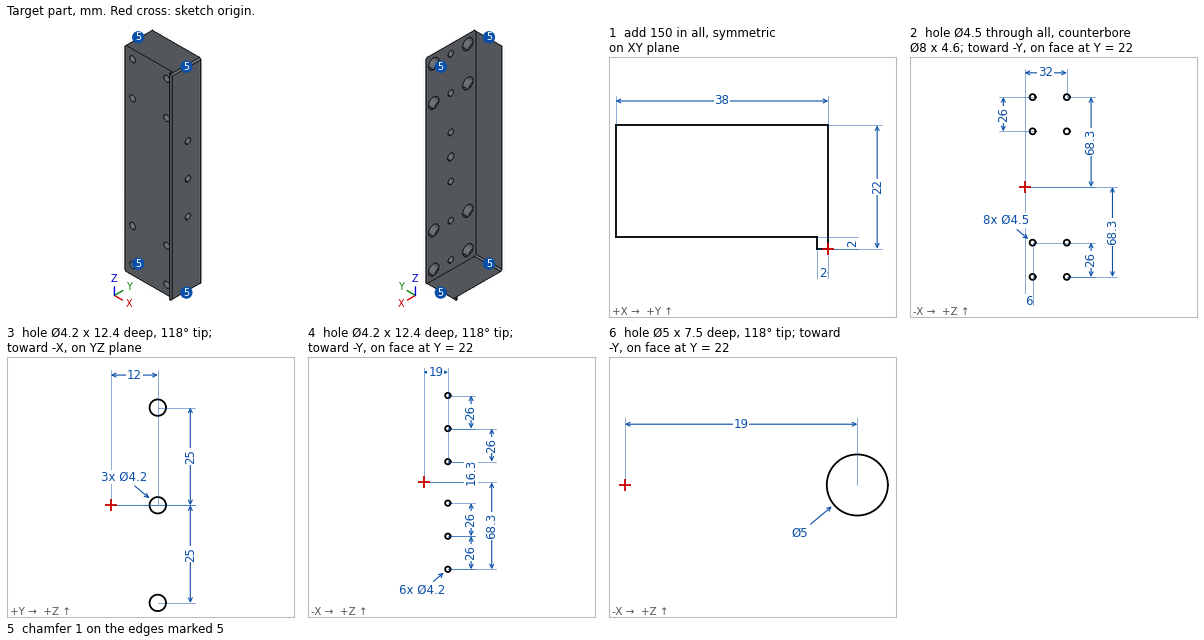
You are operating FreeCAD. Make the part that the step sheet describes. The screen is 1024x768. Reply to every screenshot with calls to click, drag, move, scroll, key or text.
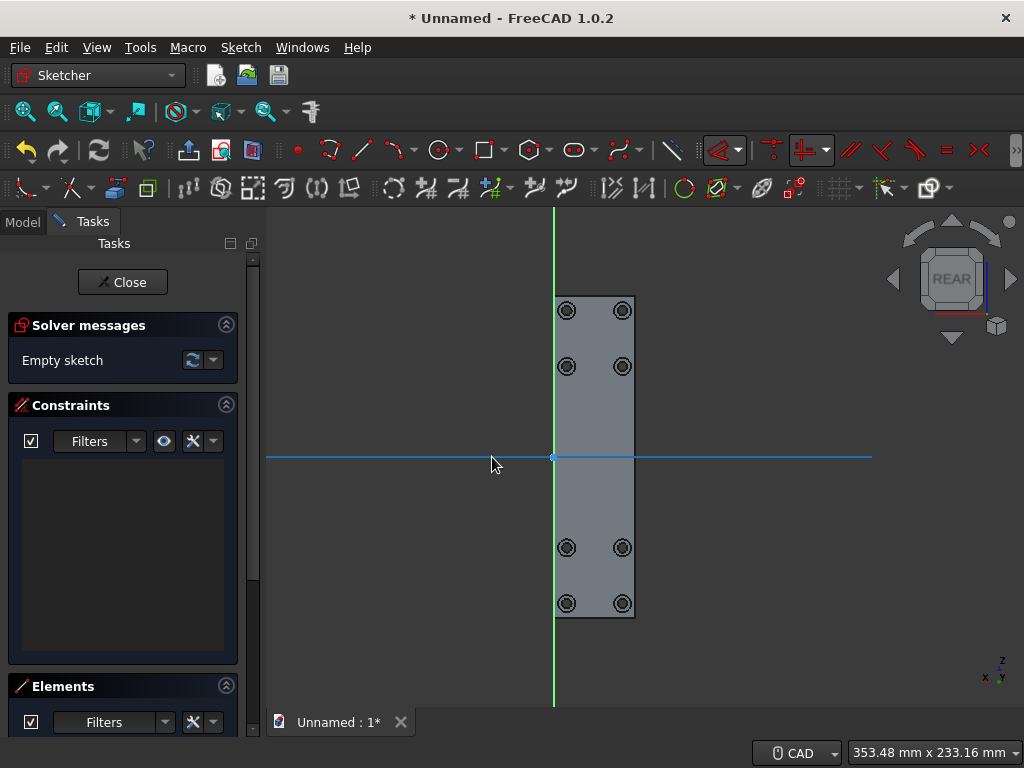
click(440, 150)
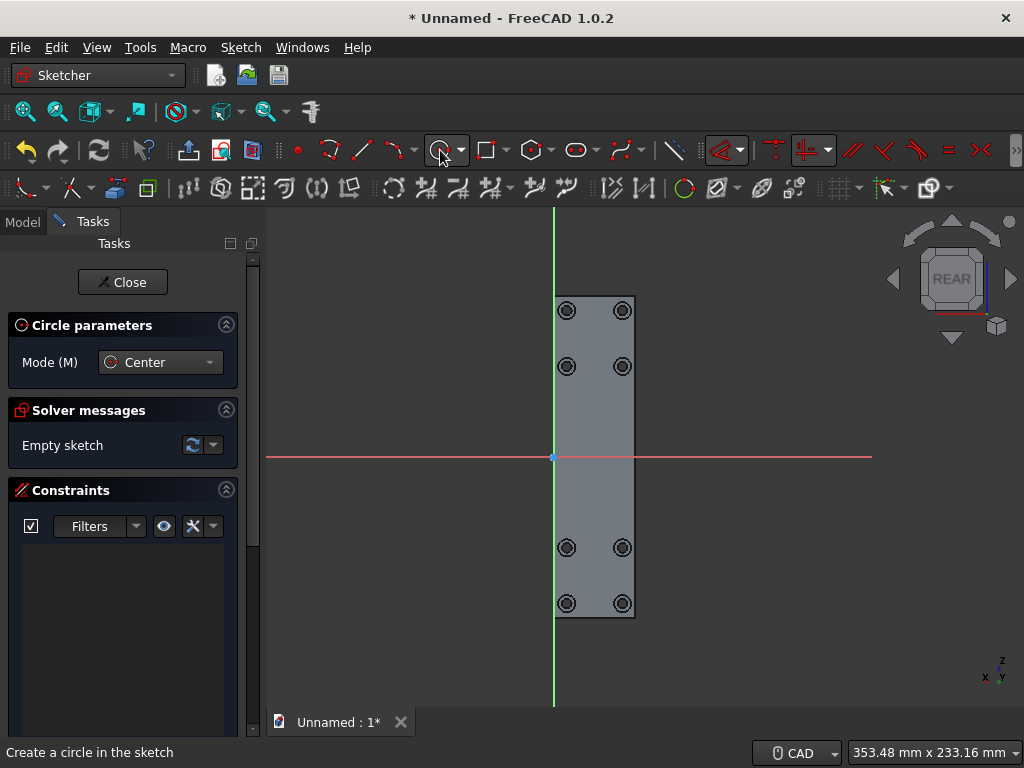
scroll(595, 422, up, 9)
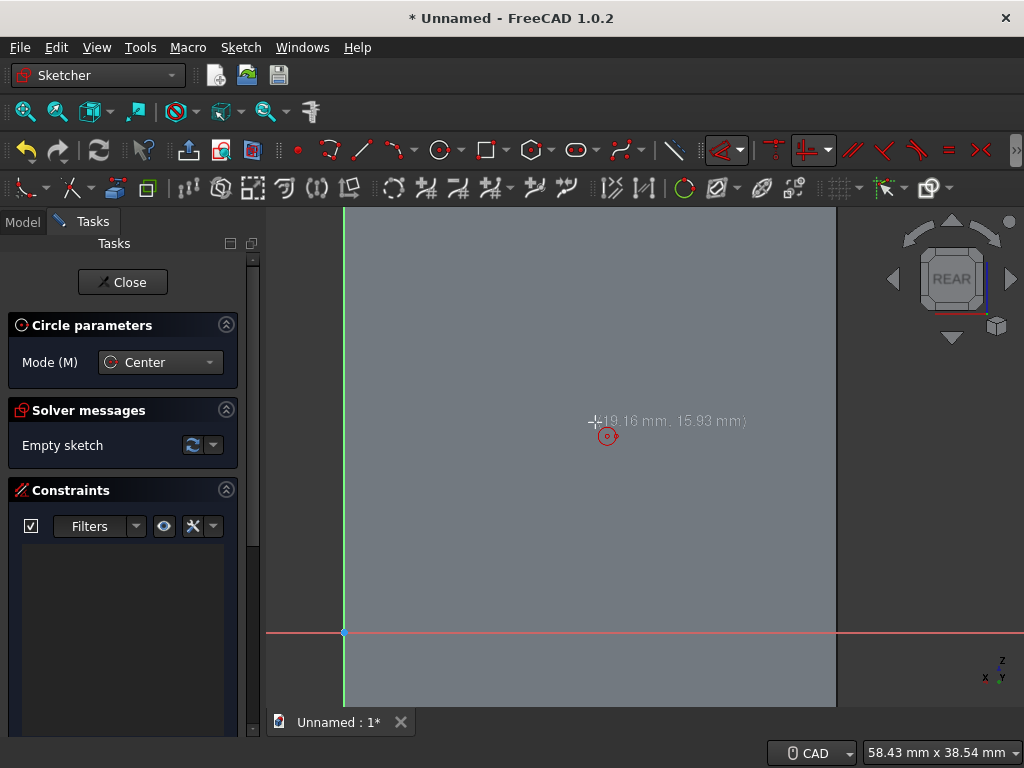
scroll(595, 422, down, 9)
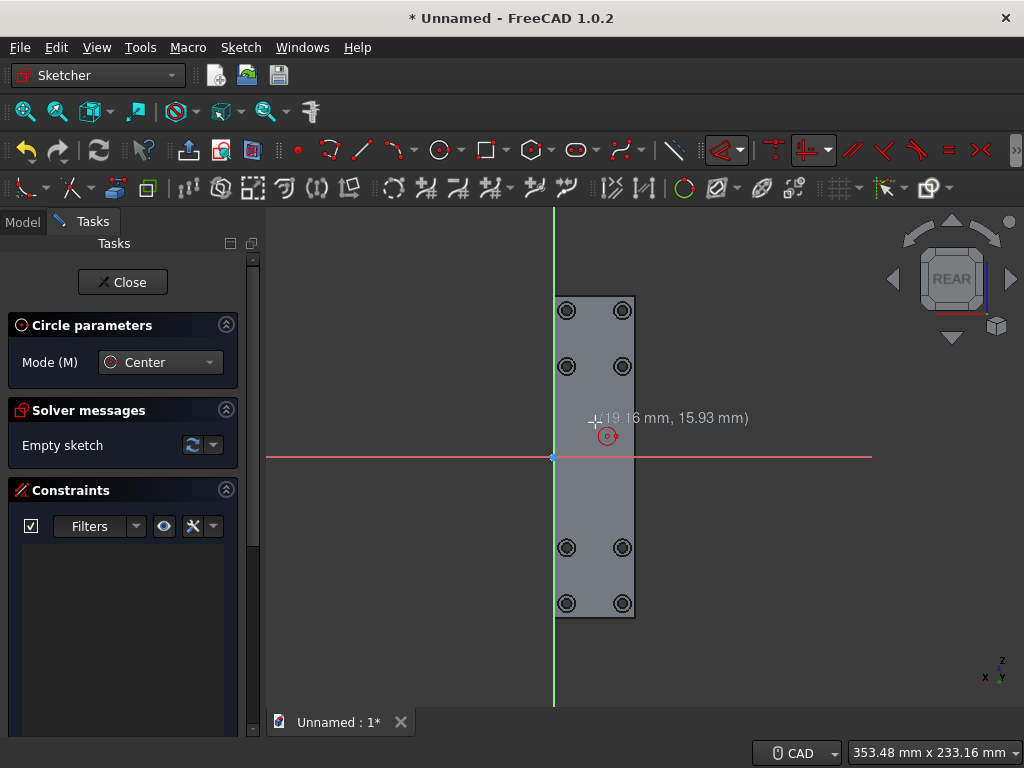
click(595, 422)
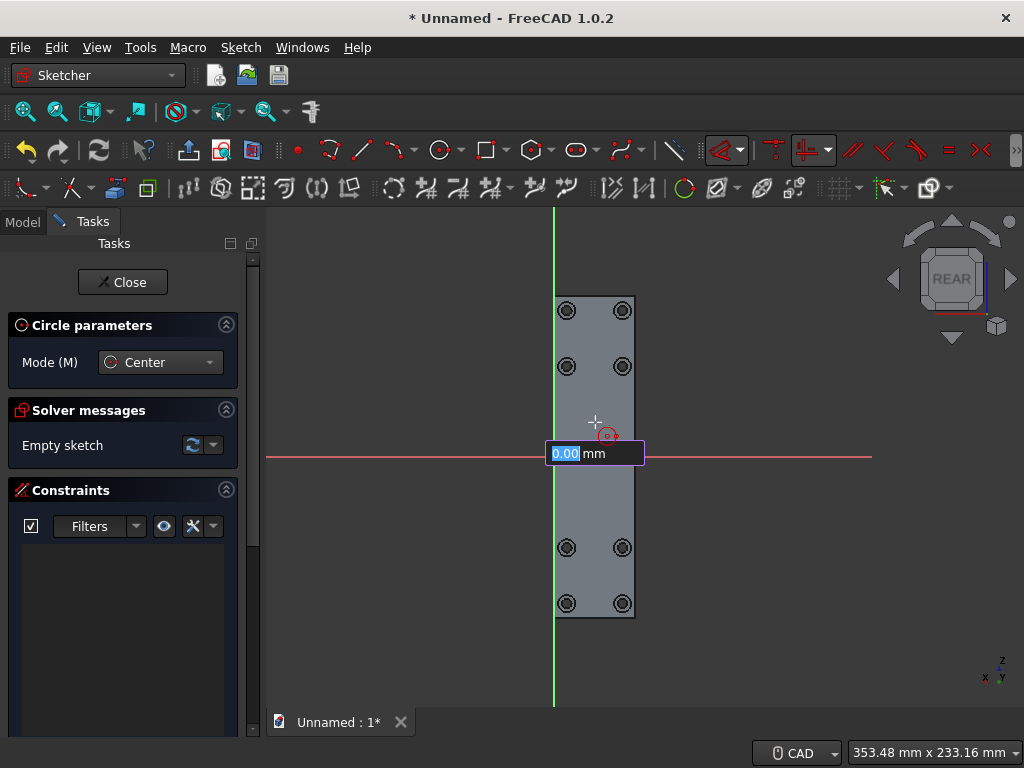
scroll(598, 419, up, 7)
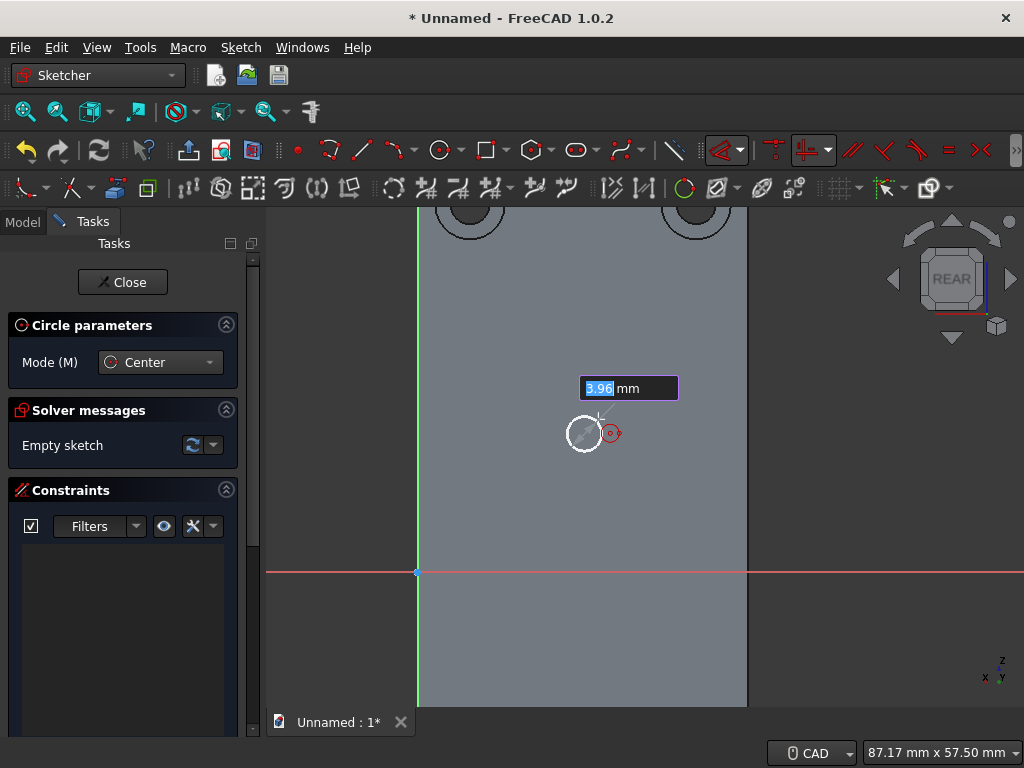
click(596, 418)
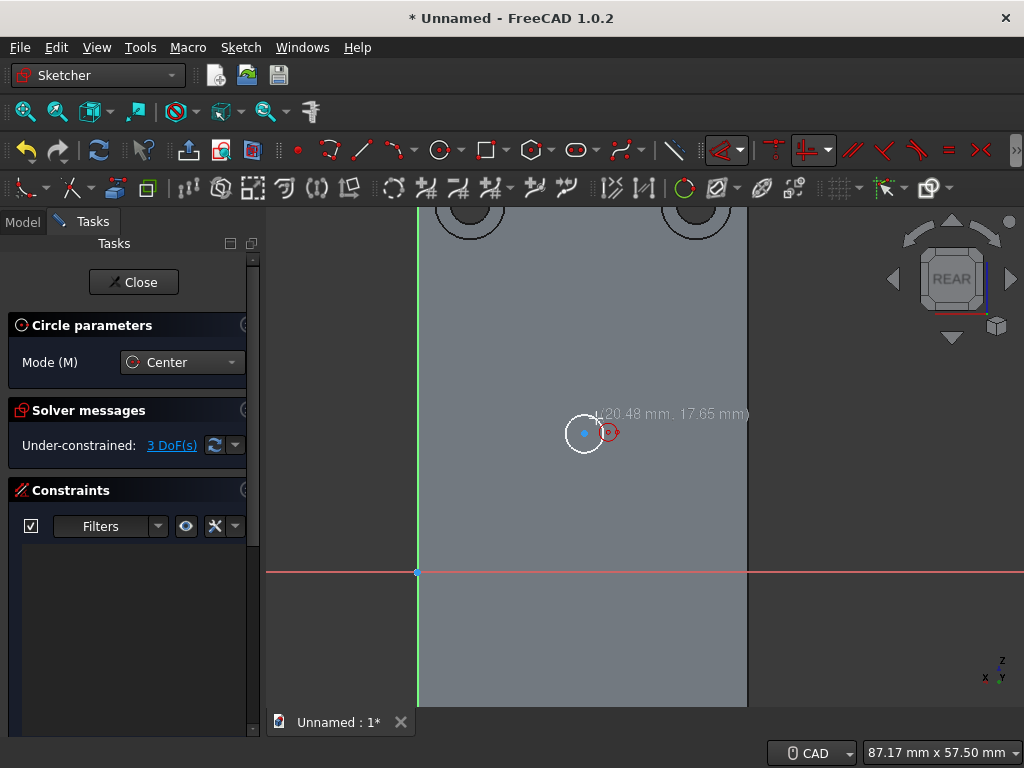
scroll(598, 419, down, 7)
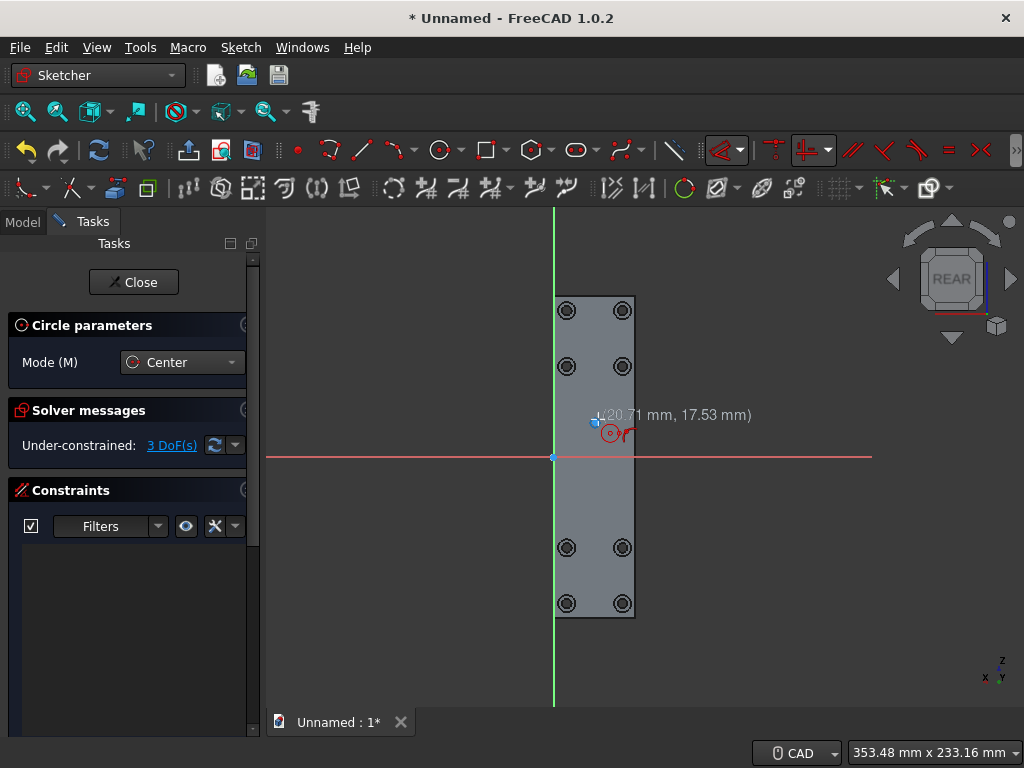
scroll(595, 604, up, 9)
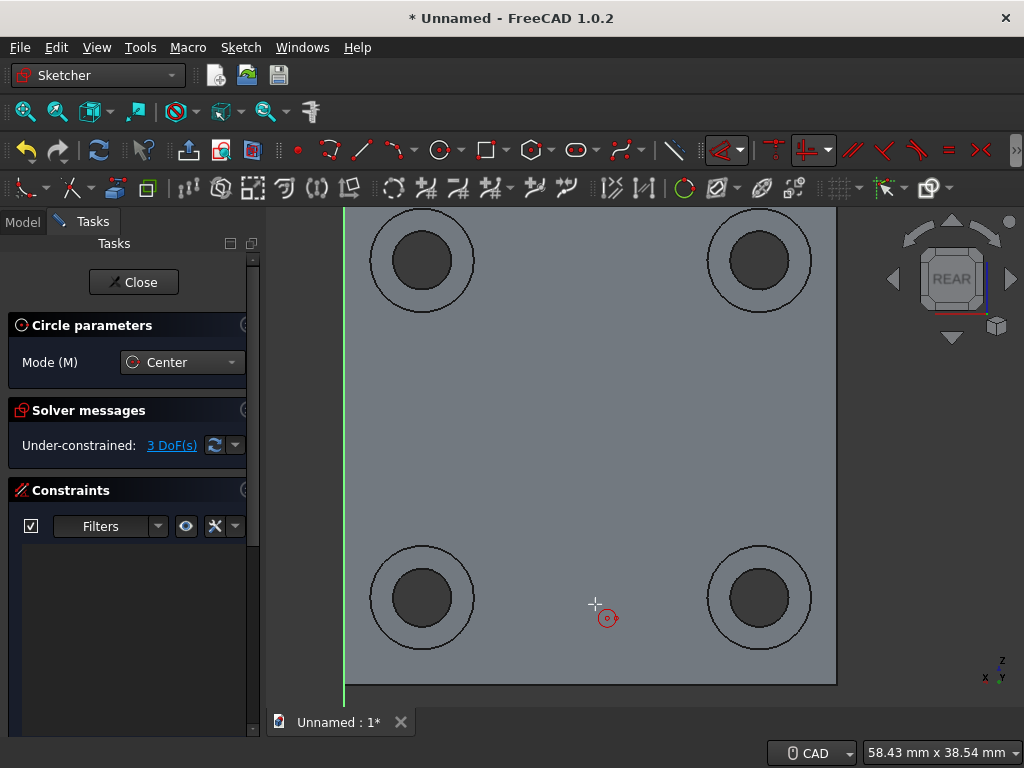
scroll(595, 605, down, 9)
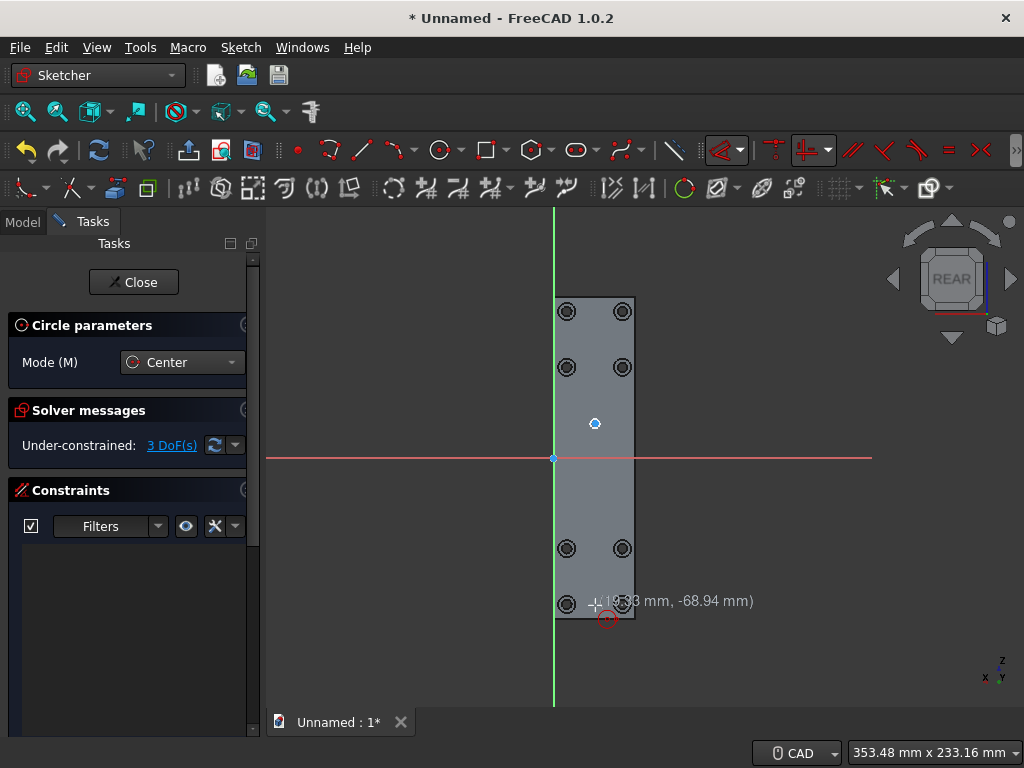
click(595, 604)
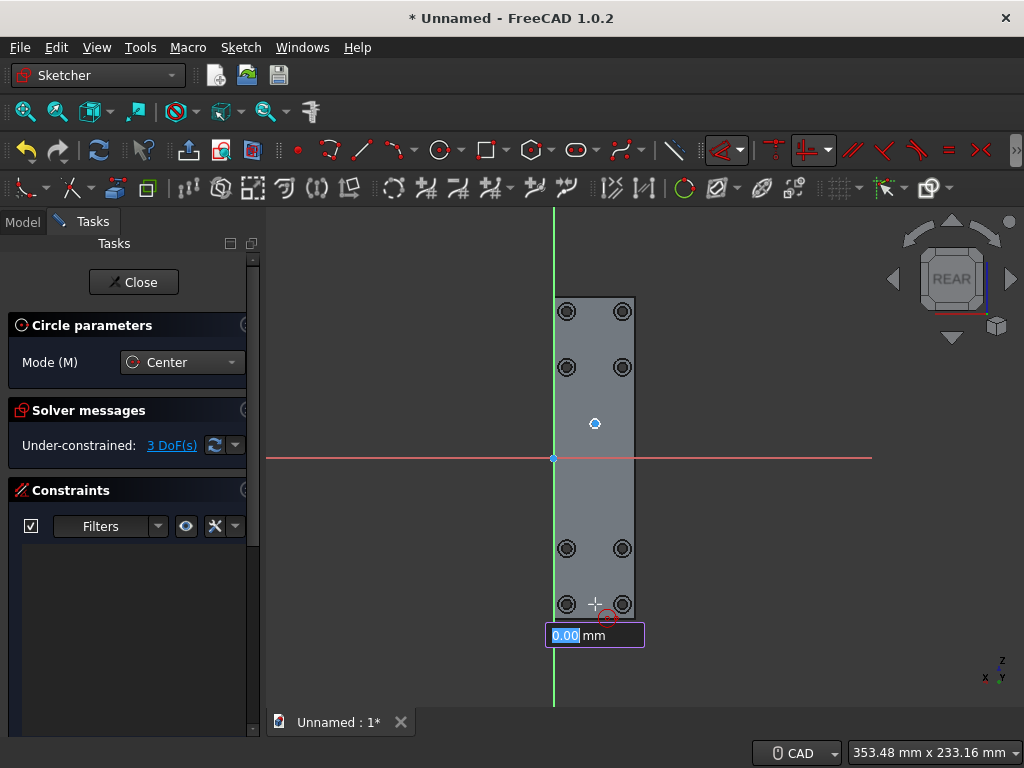
scroll(598, 601, up, 7)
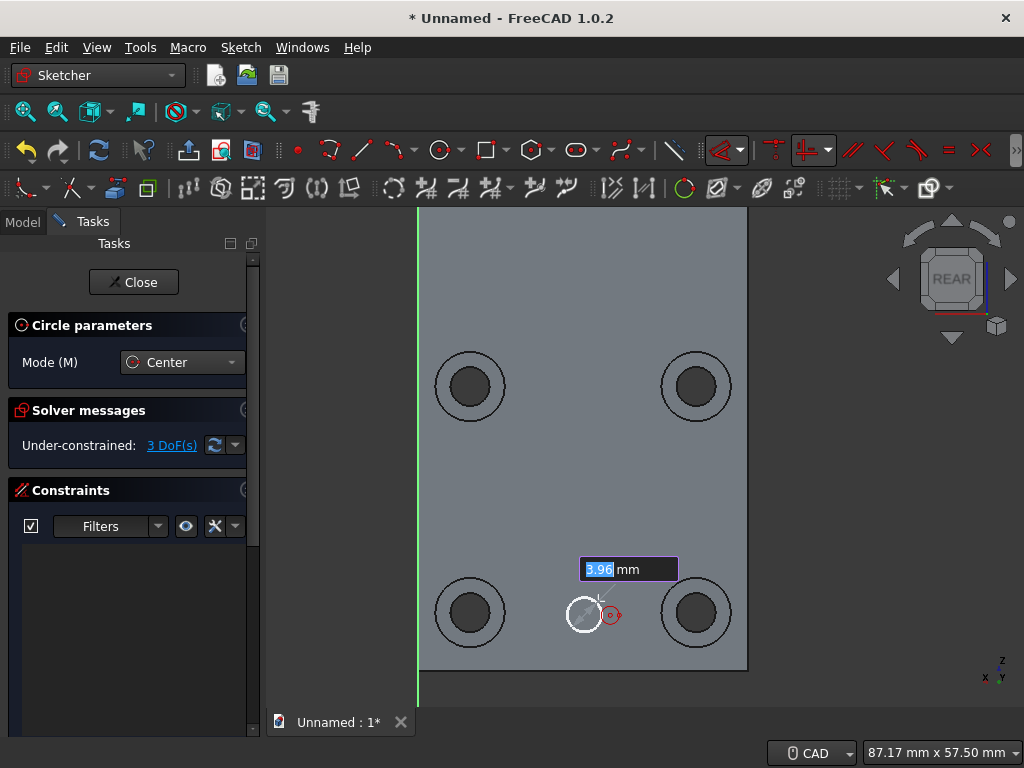
click(596, 600)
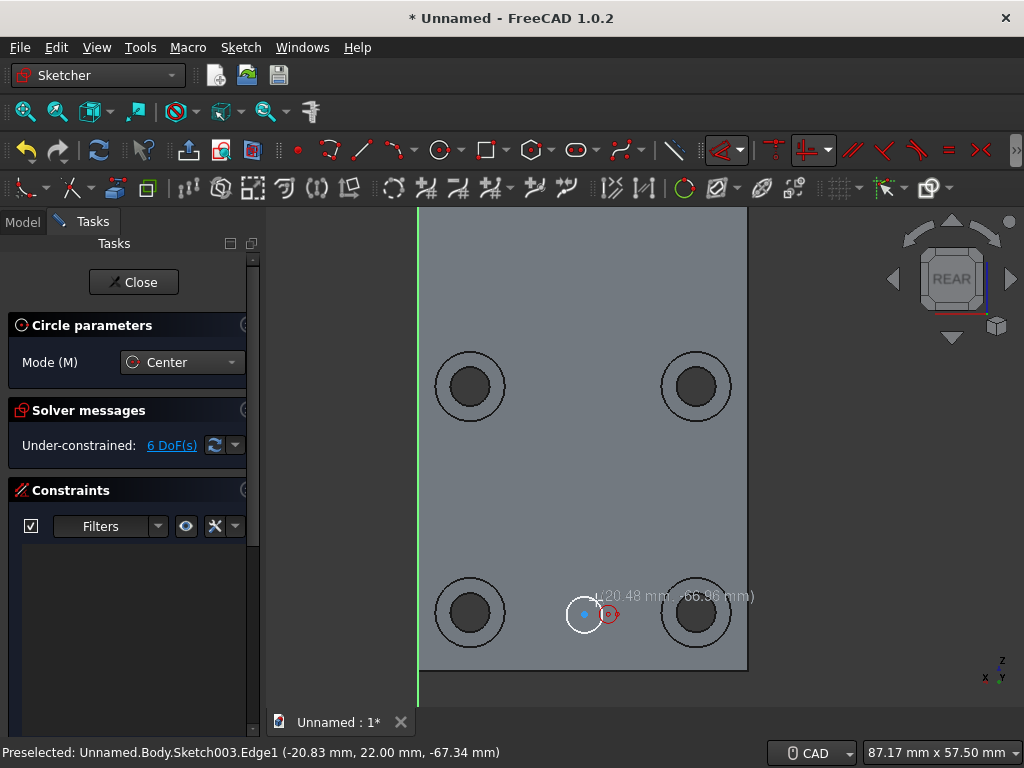
scroll(583, 387, up, 2)